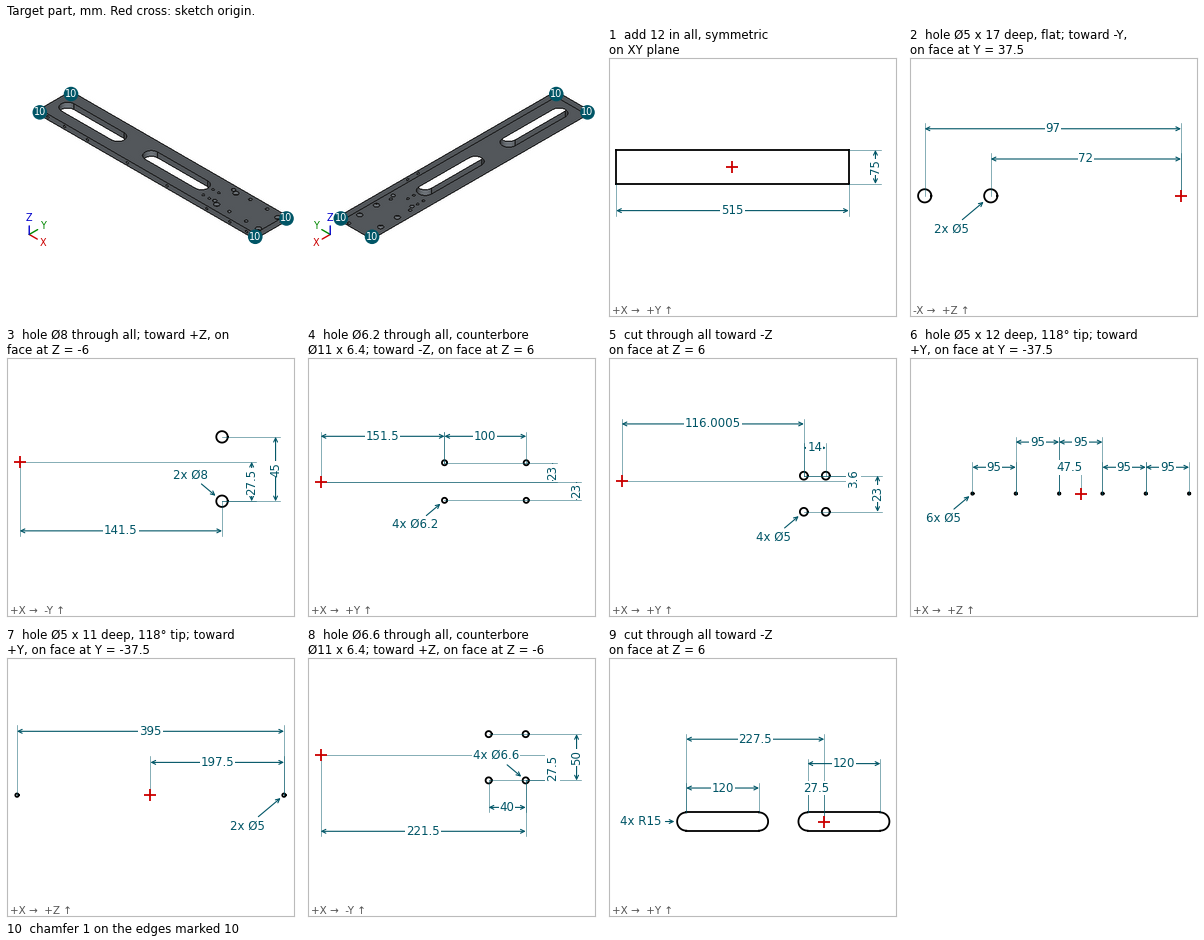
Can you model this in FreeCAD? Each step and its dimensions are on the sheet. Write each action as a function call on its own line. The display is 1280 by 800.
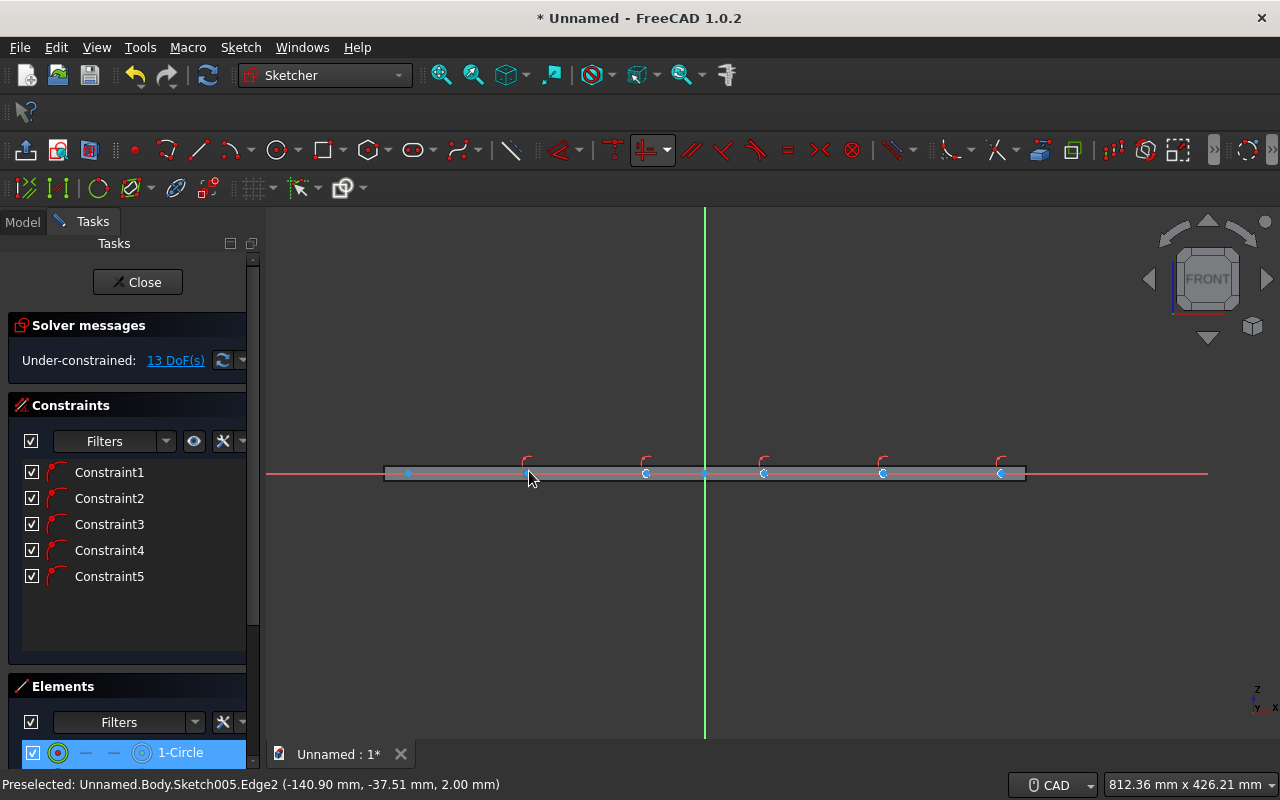
scroll(648, 471, up, 9)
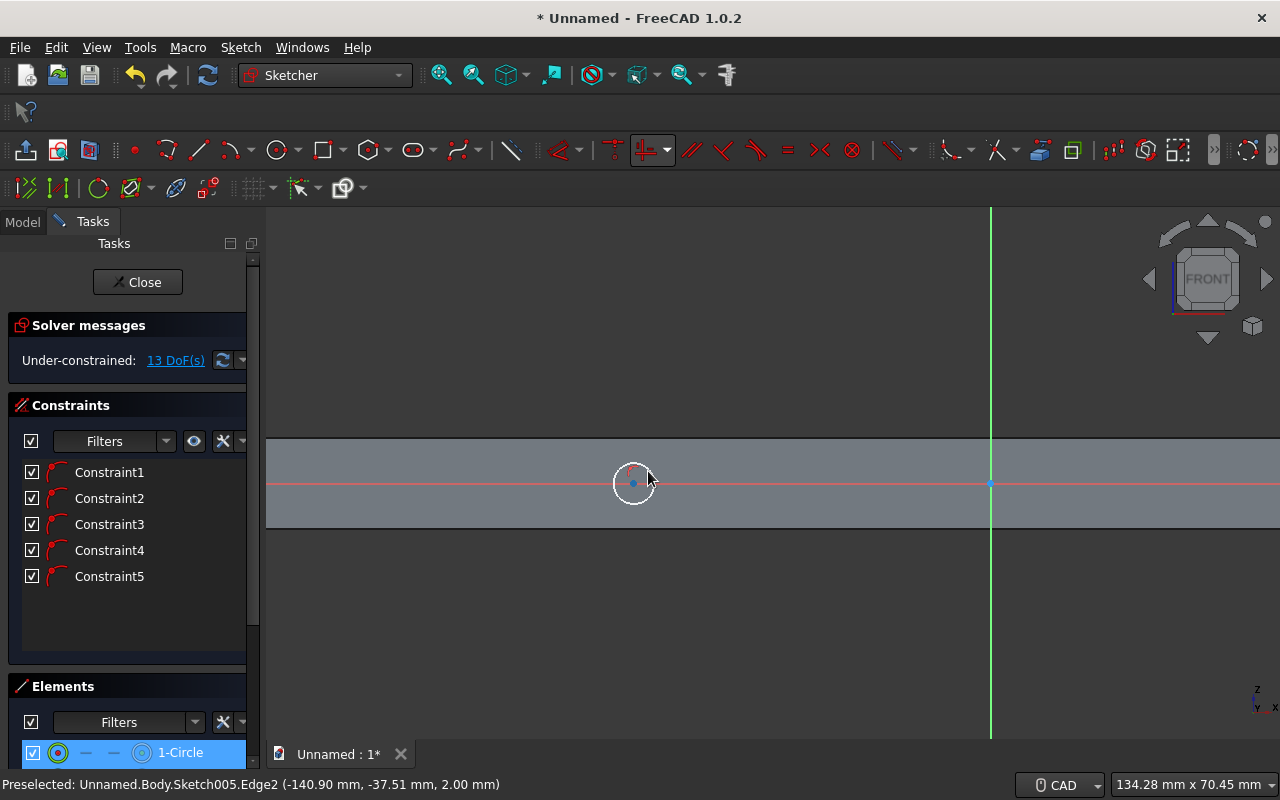
click(648, 469)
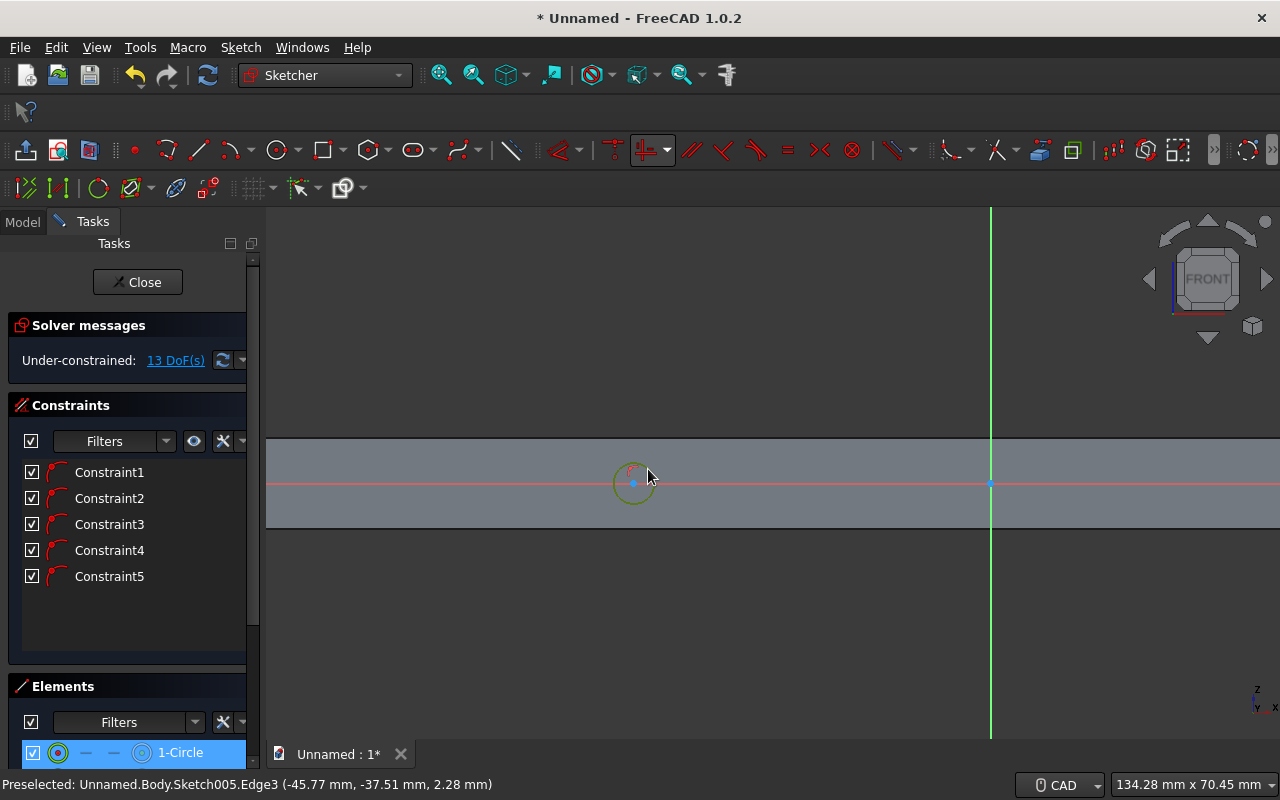
scroll(648, 471, down, 9)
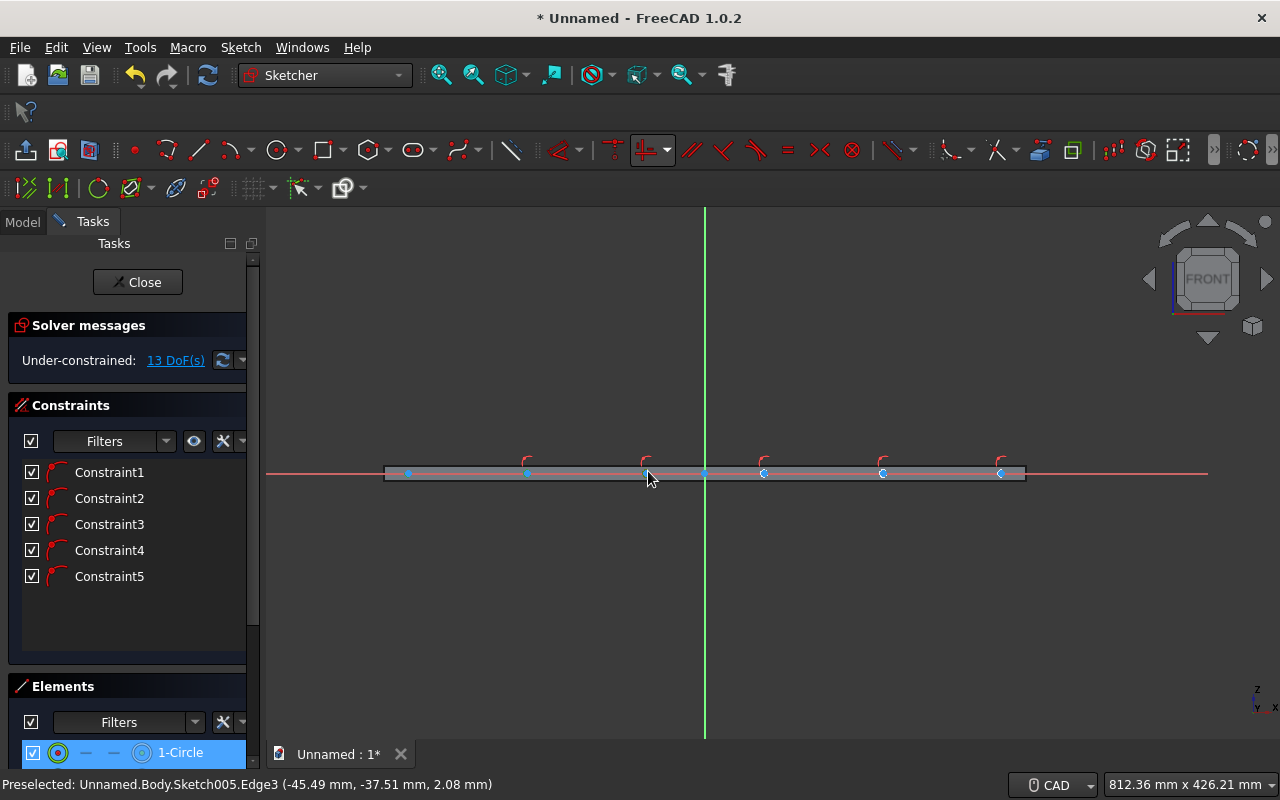
scroll(766, 471, up, 9)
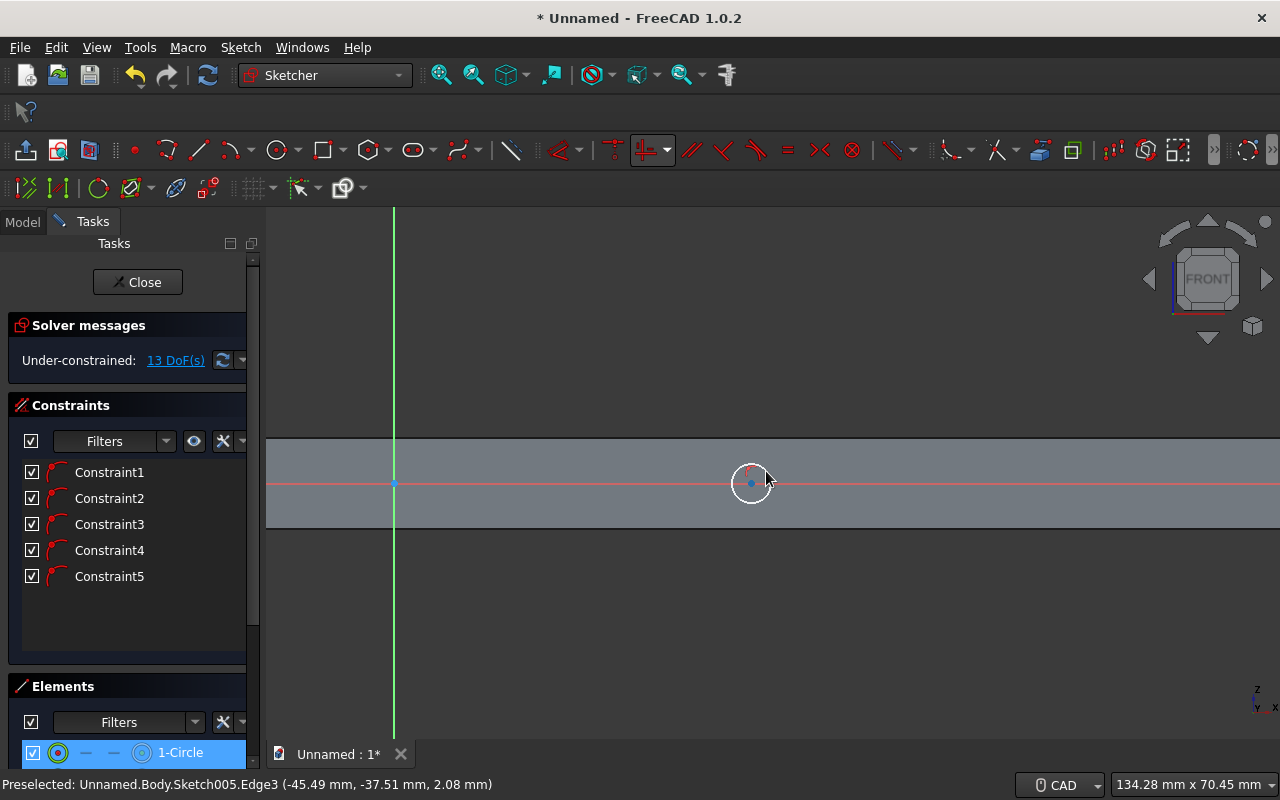
click(765, 470)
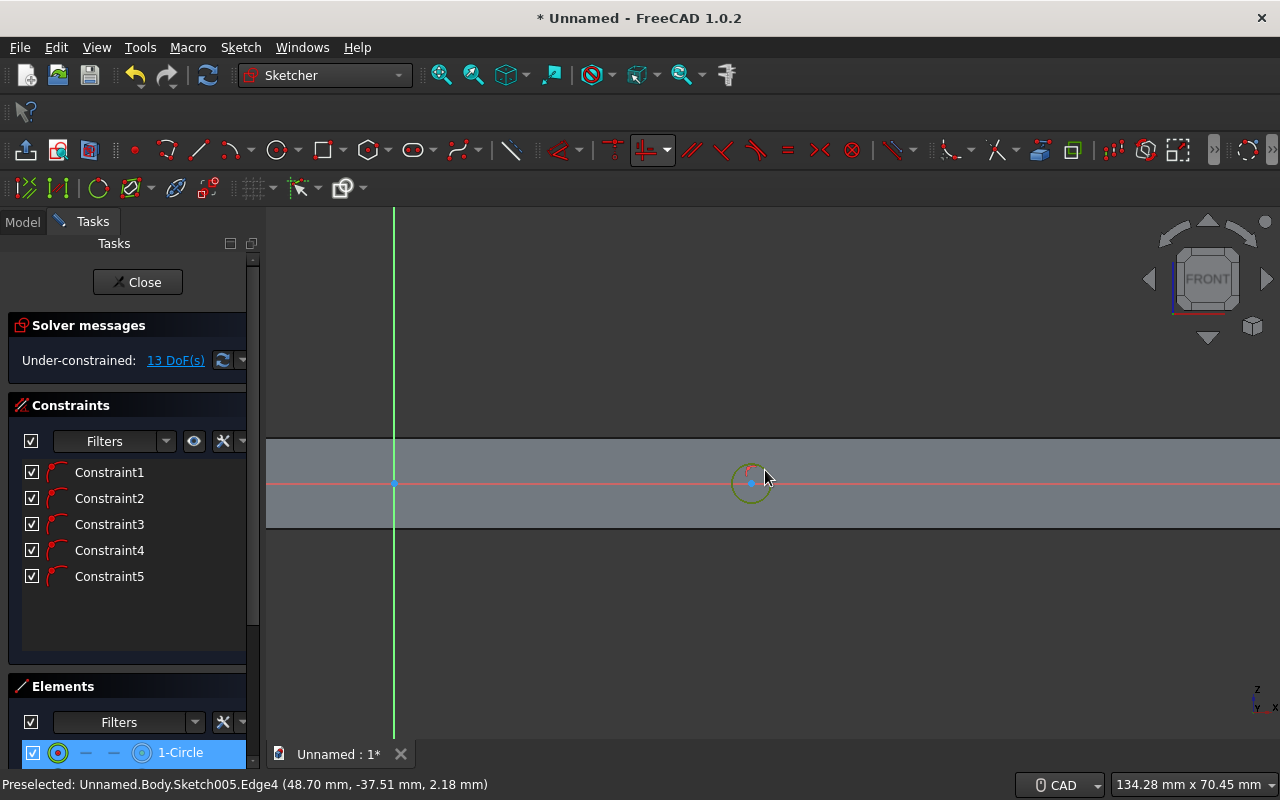
scroll(766, 471, down, 9)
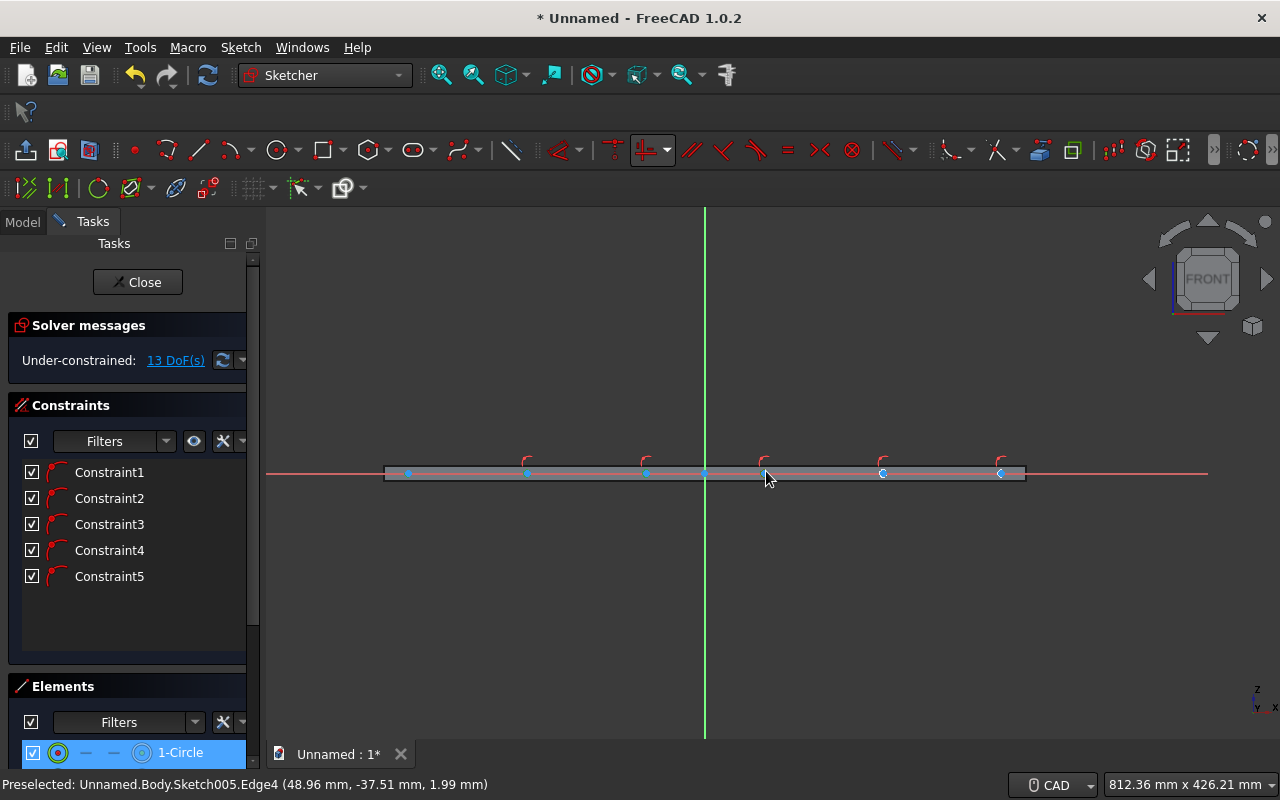
scroll(885, 471, up, 9)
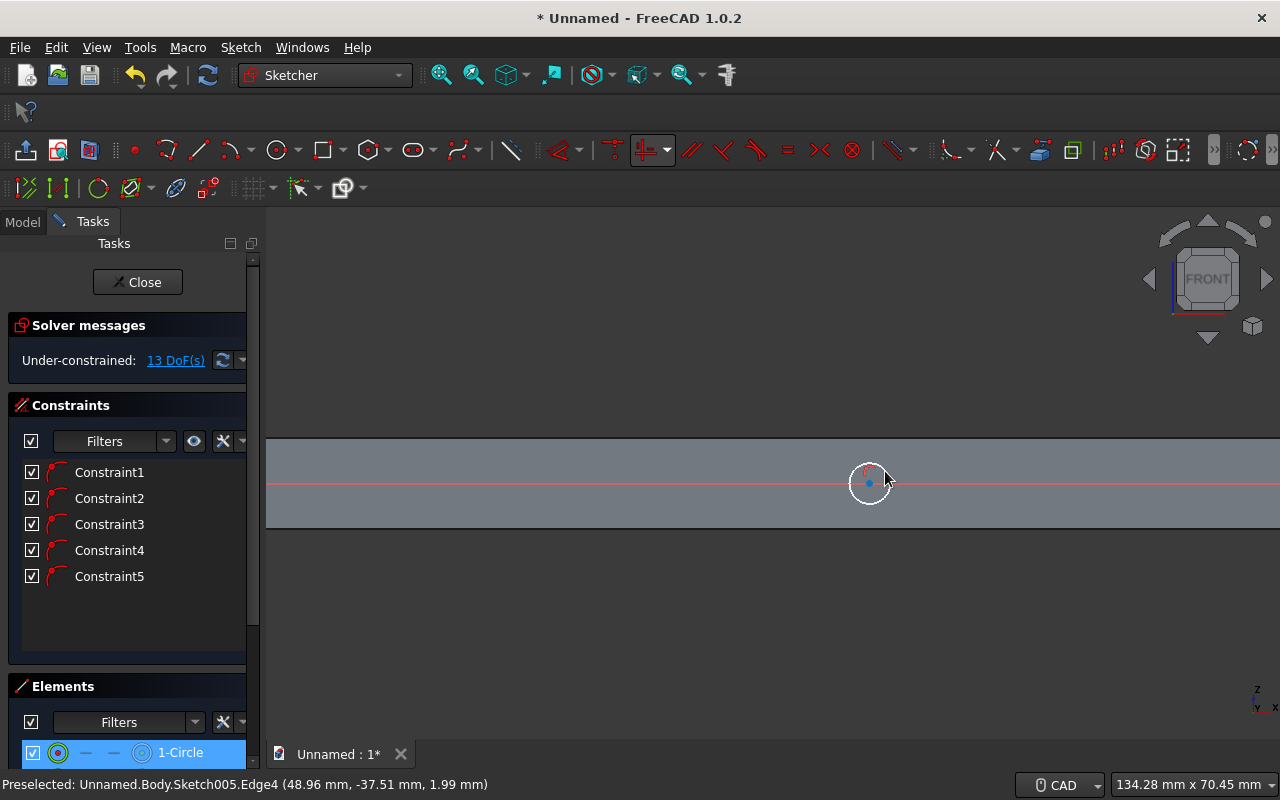
click(884, 469)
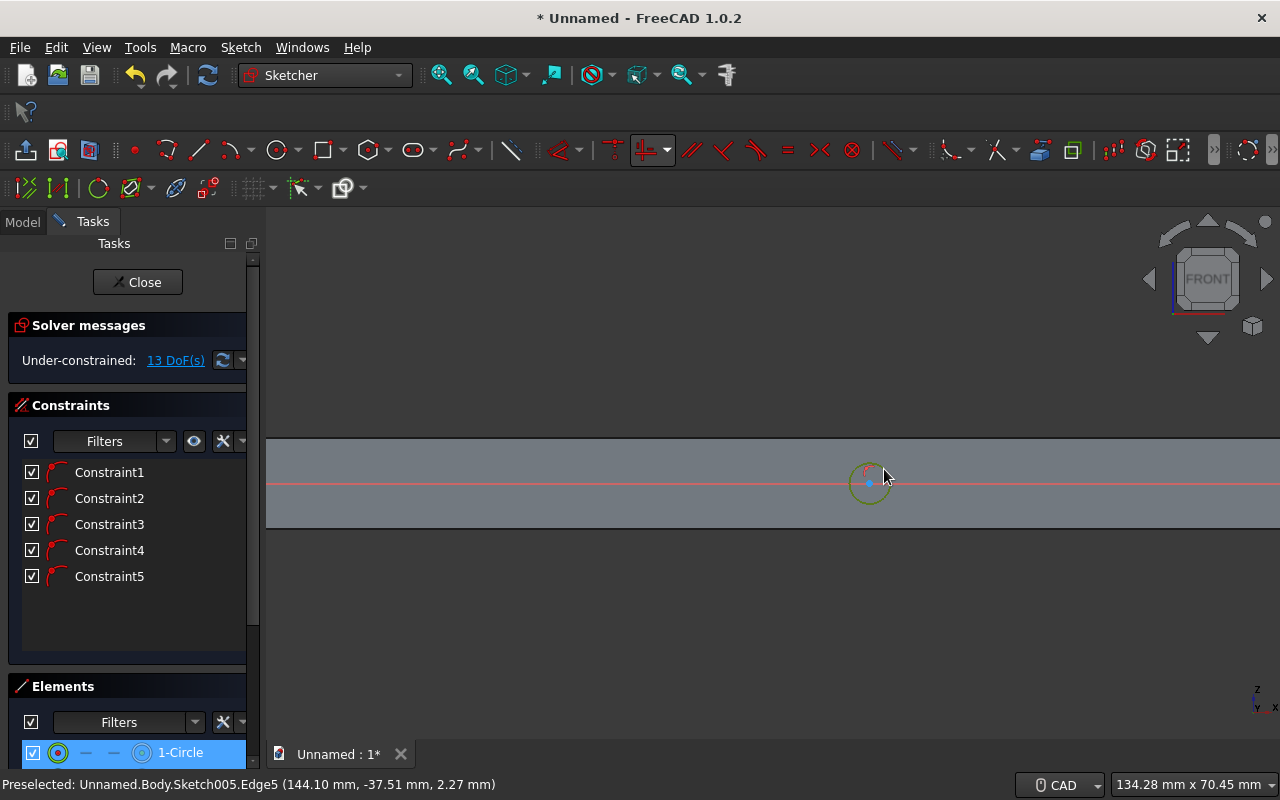
scroll(885, 471, down, 9)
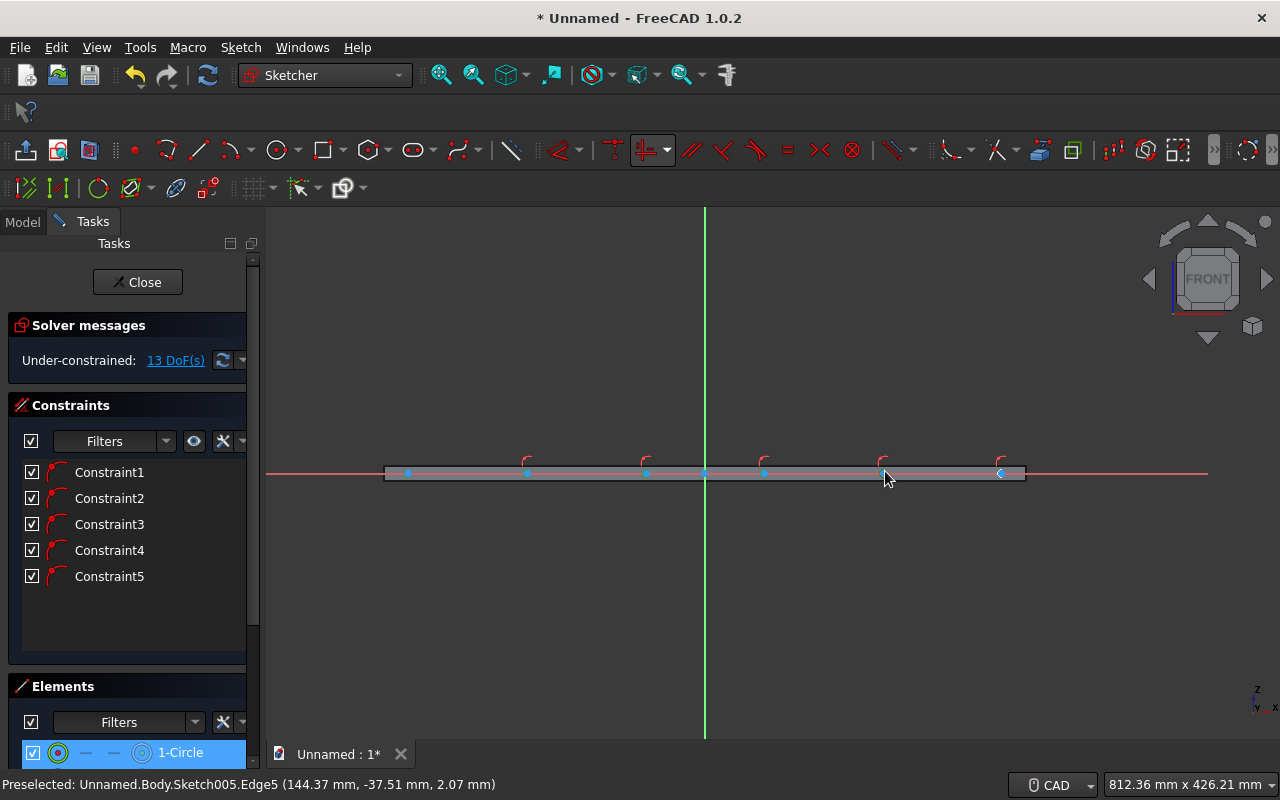
scroll(1003, 471, up, 10)